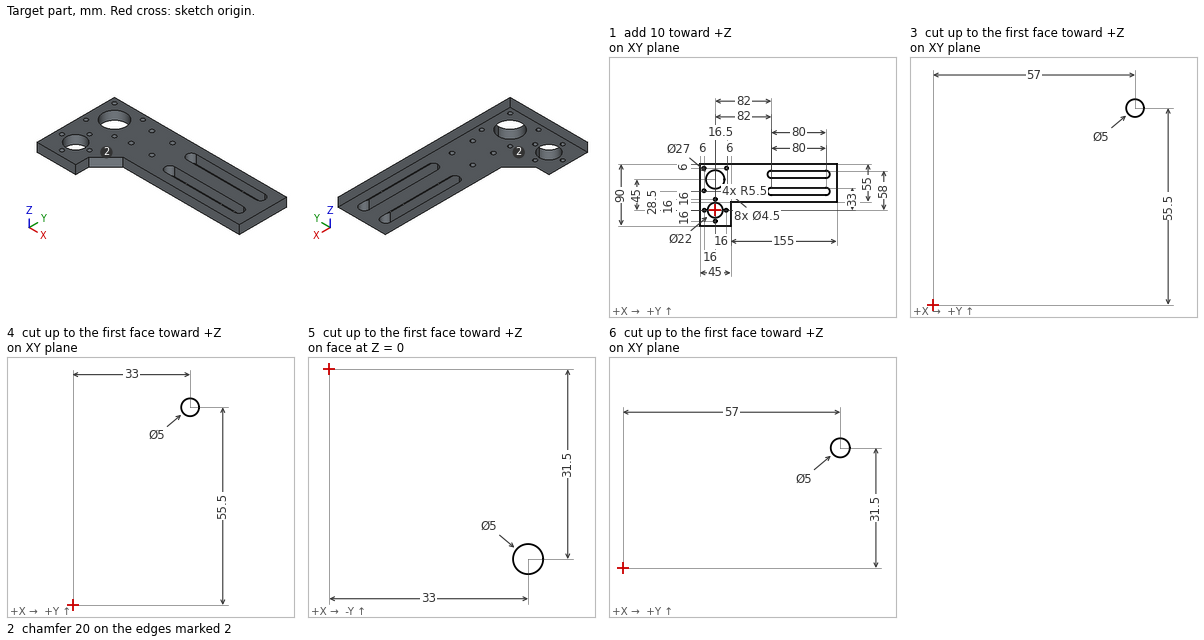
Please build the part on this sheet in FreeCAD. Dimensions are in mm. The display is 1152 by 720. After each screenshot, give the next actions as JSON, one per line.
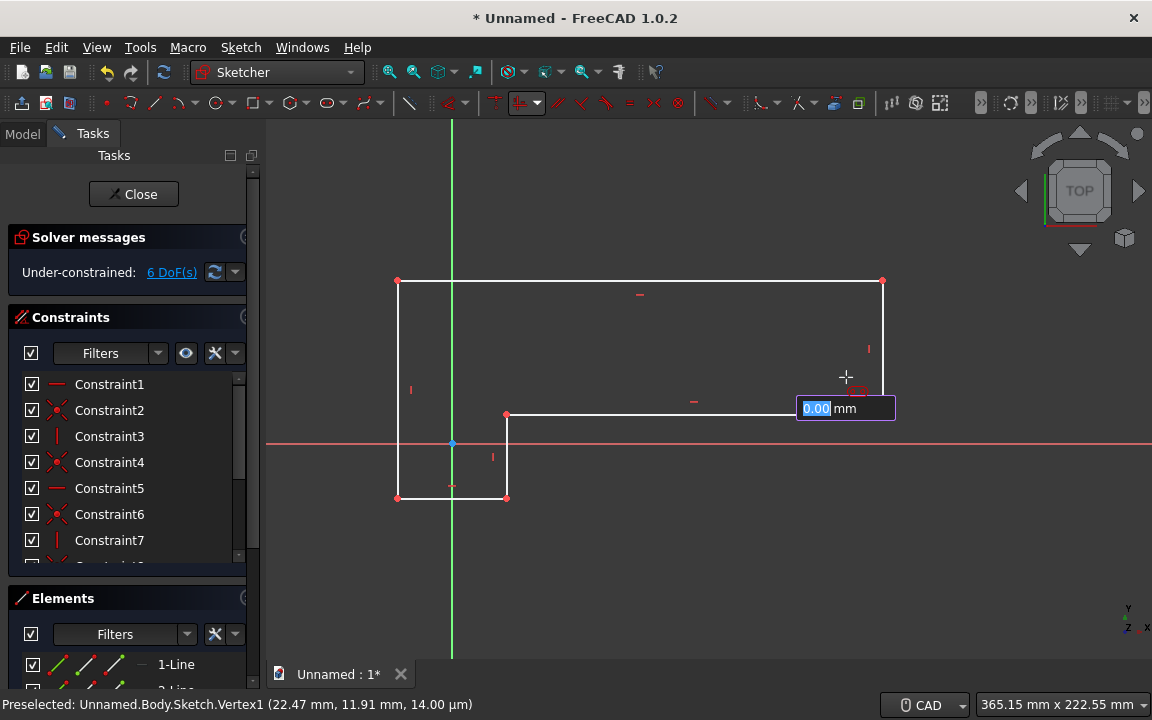
{"action": "left_click", "coordinate": [749, 391]}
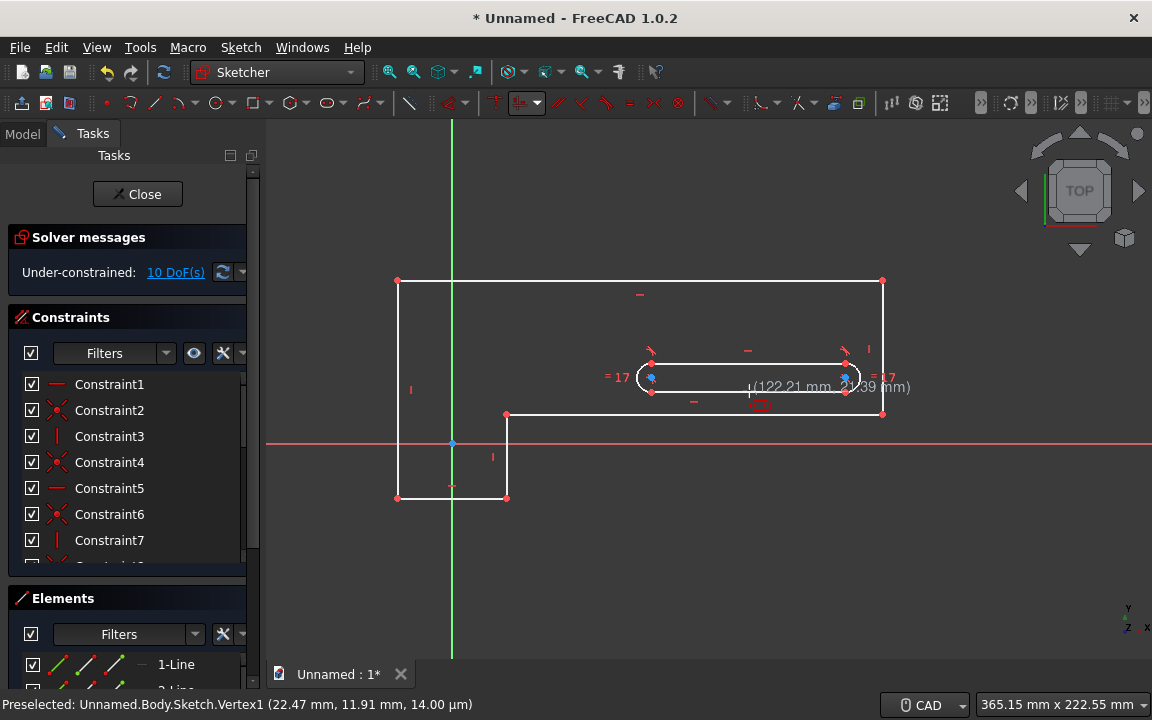
{"action": "scroll", "coordinate": [651, 317], "scroll_direction": "up", "scroll_amount": 3}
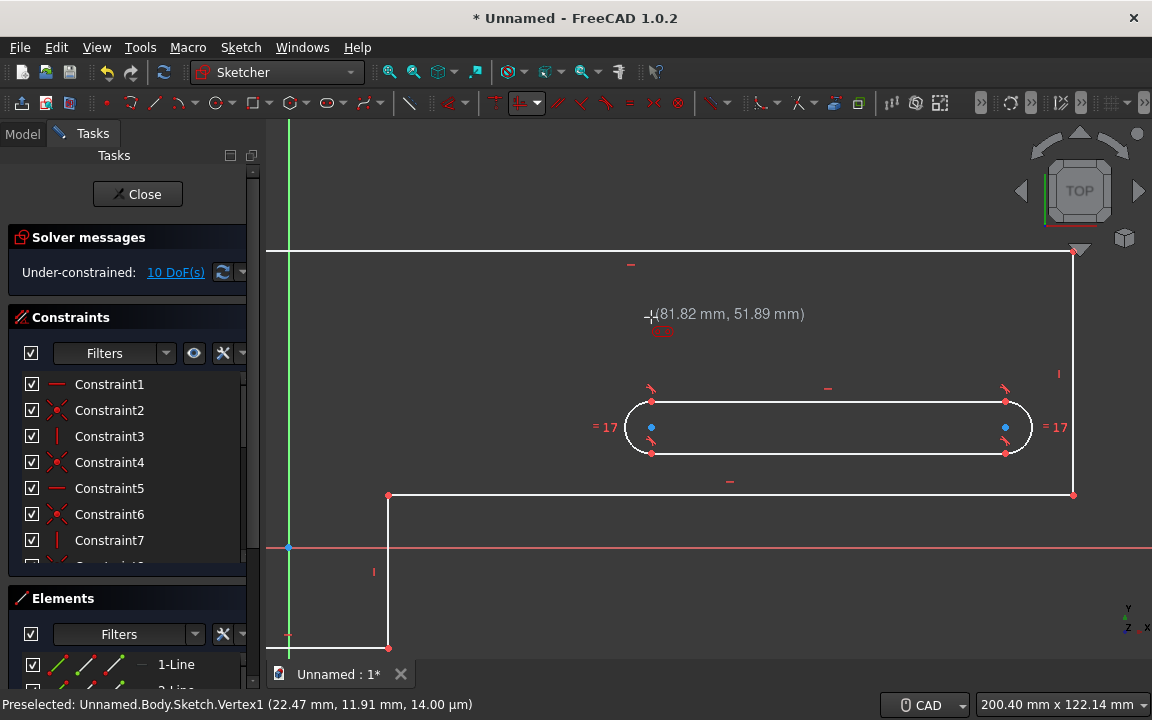
{"action": "left_click", "coordinate": [651, 316]}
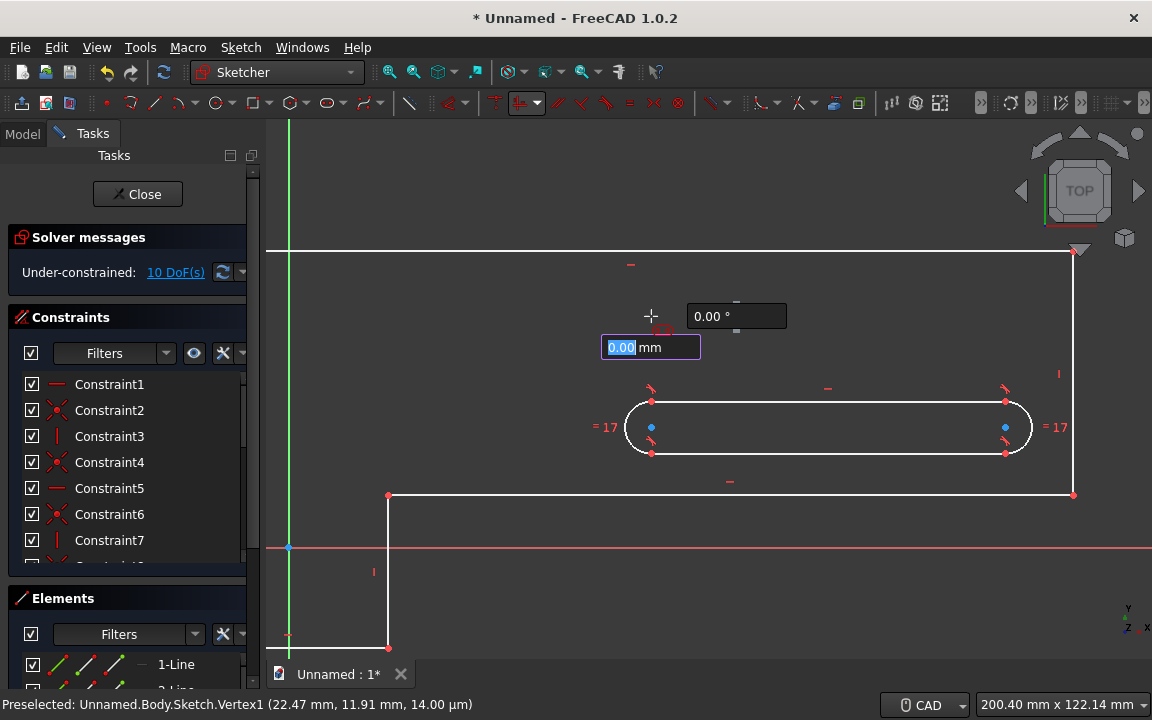
{"action": "scroll", "coordinate": [651, 317], "scroll_direction": "down", "scroll_amount": 3}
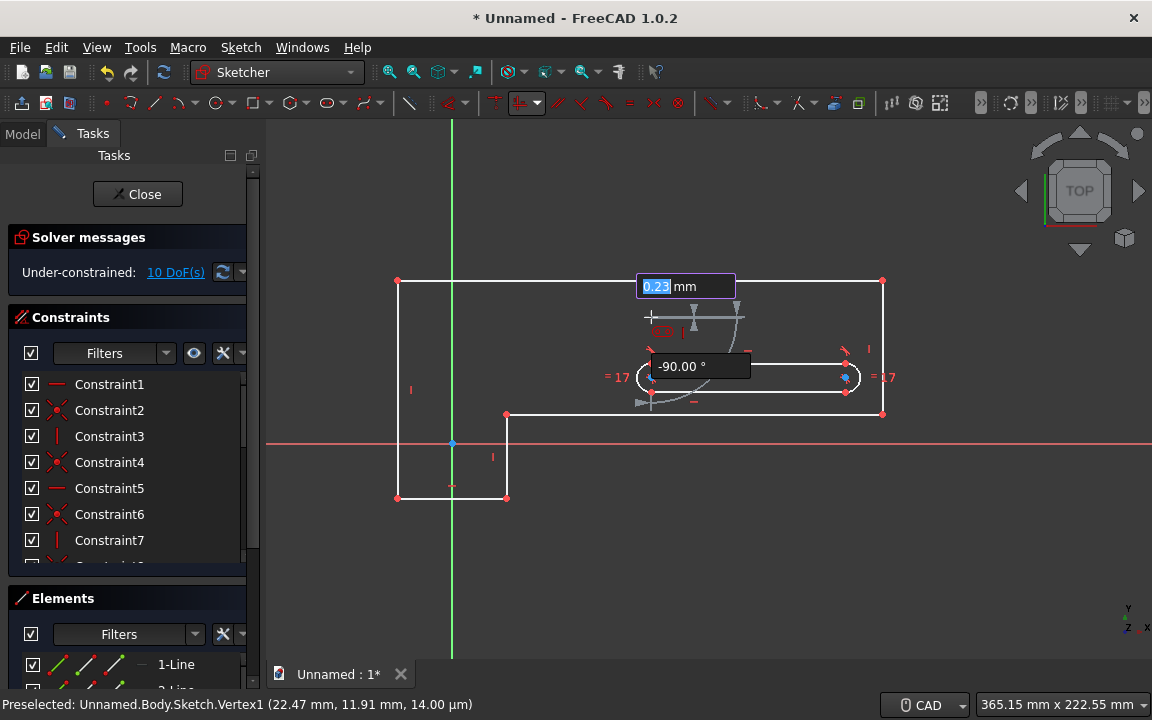
{"action": "left_click", "coordinate": [846, 317]}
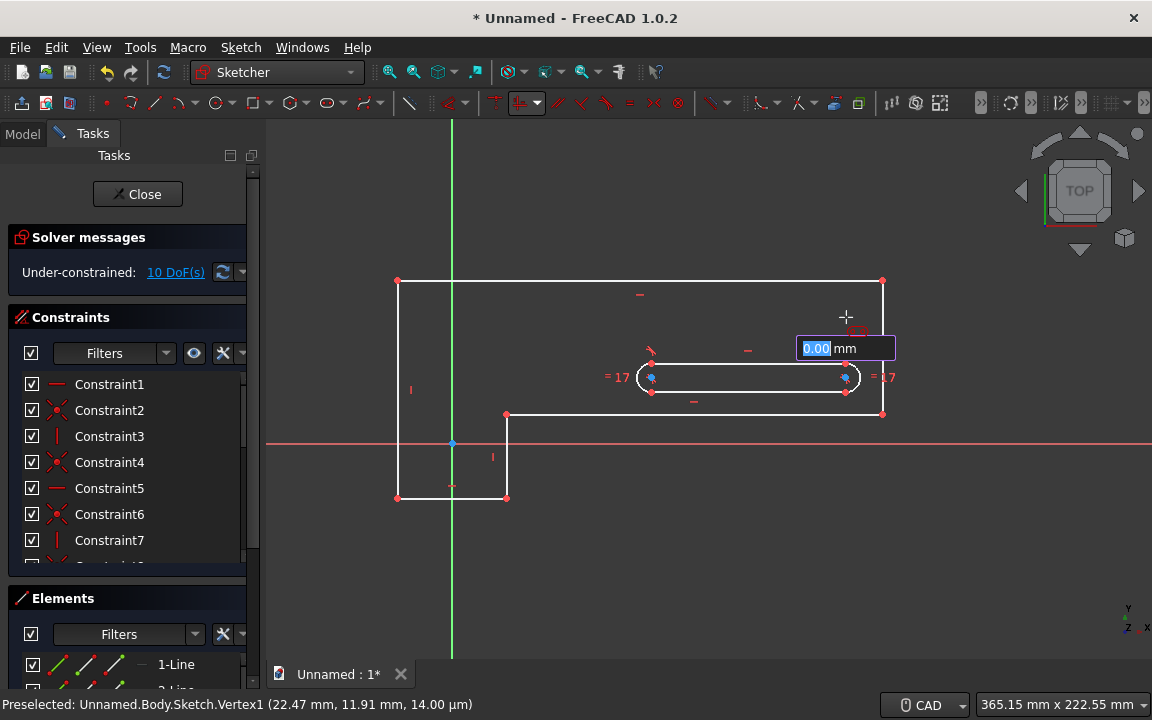
{"action": "left_click", "coordinate": [749, 330]}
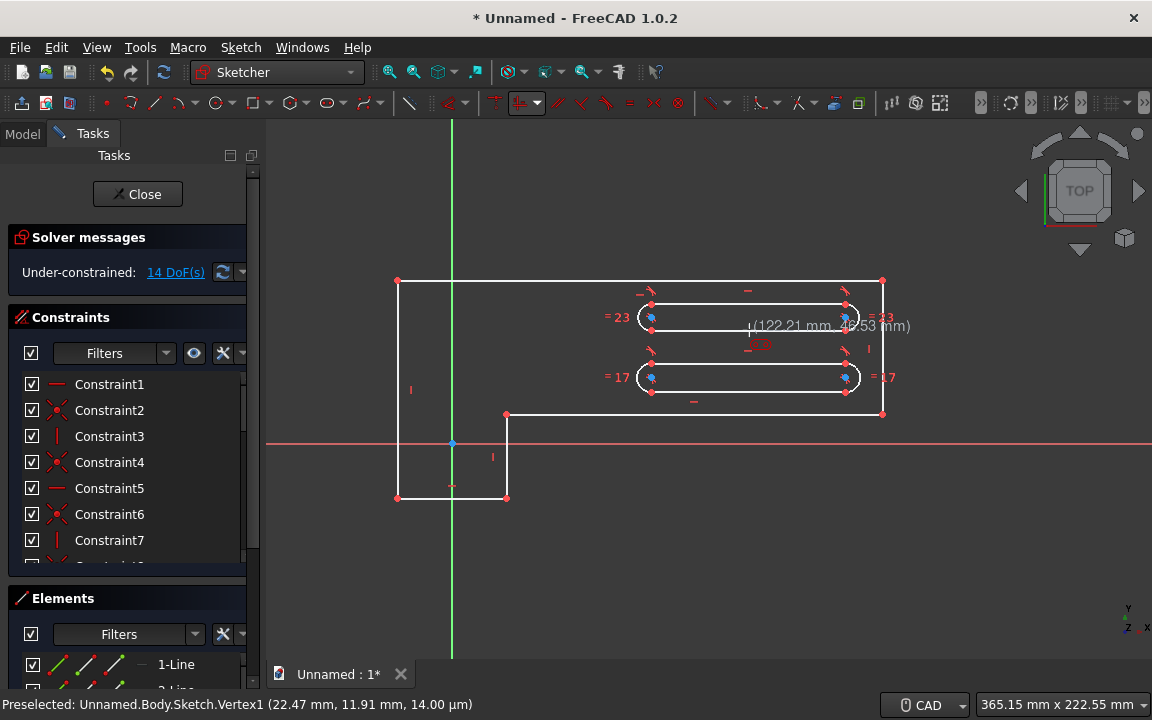
{"action": "key", "text": "g c"}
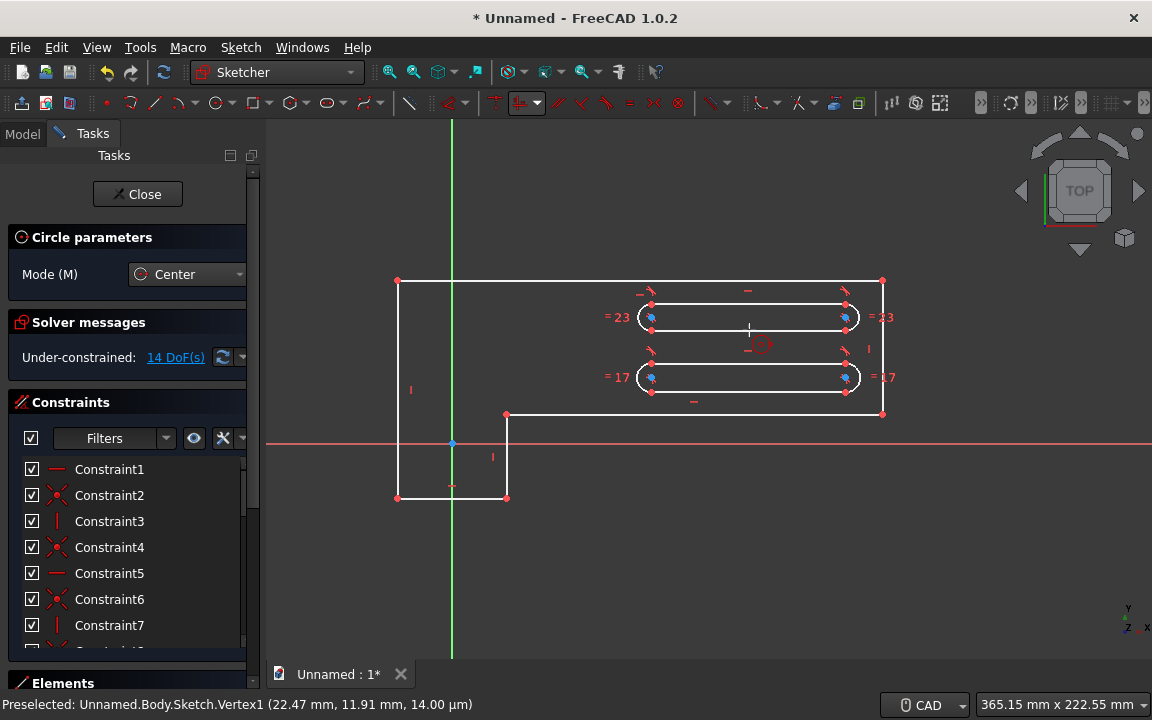
{"action": "scroll", "coordinate": [452, 483], "scroll_direction": "up", "scroll_amount": 8}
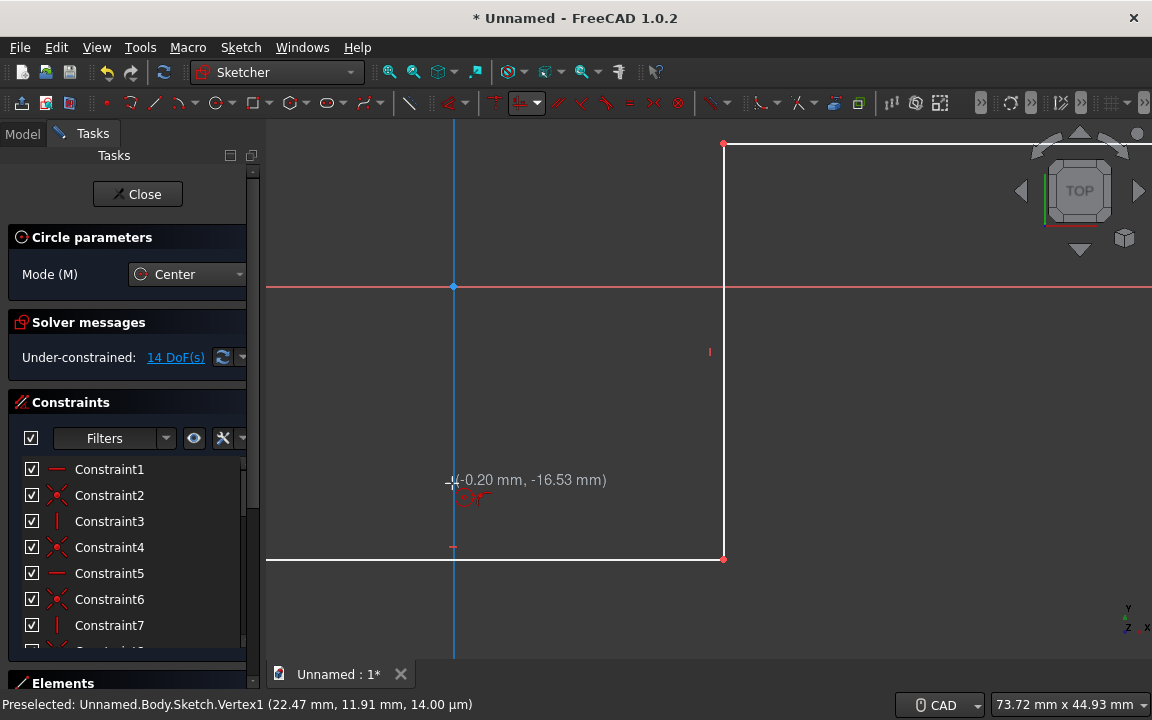
{"action": "scroll", "coordinate": [452, 483], "scroll_direction": "down", "scroll_amount": 8}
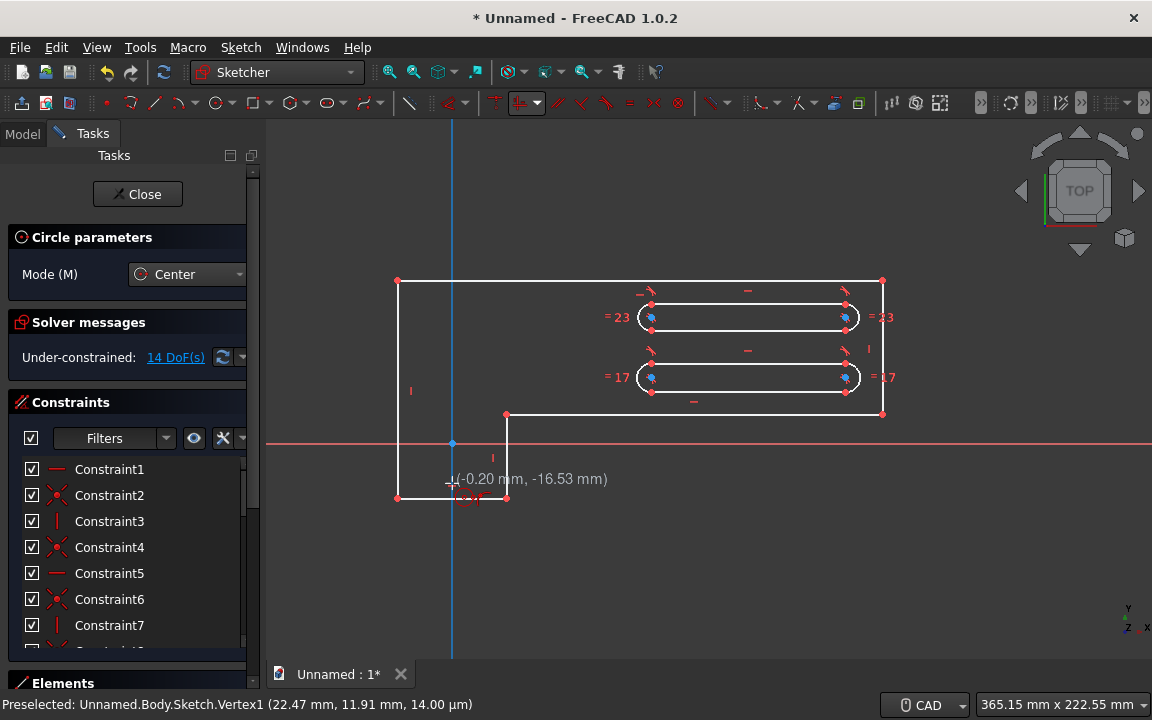
{"action": "left_click", "coordinate": [452, 483]}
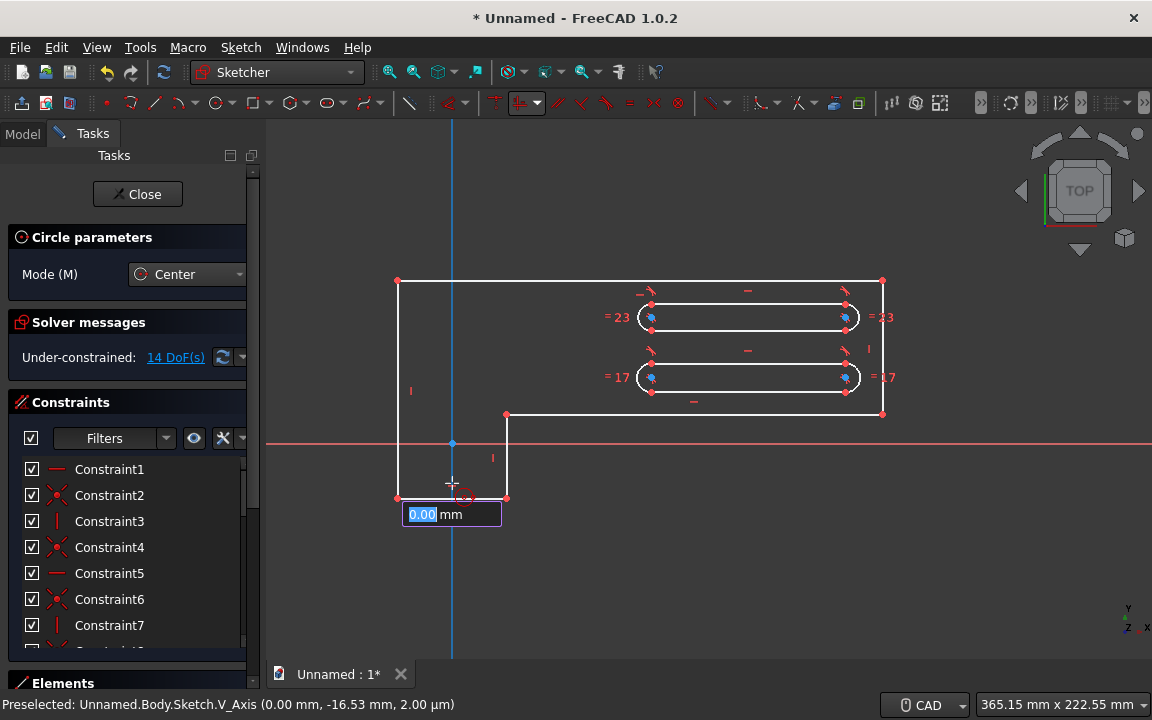
{"action": "scroll", "coordinate": [458, 481], "scroll_direction": "up", "scroll_amount": 6}
{"action": "mouse_move", "coordinate": [456, 479]}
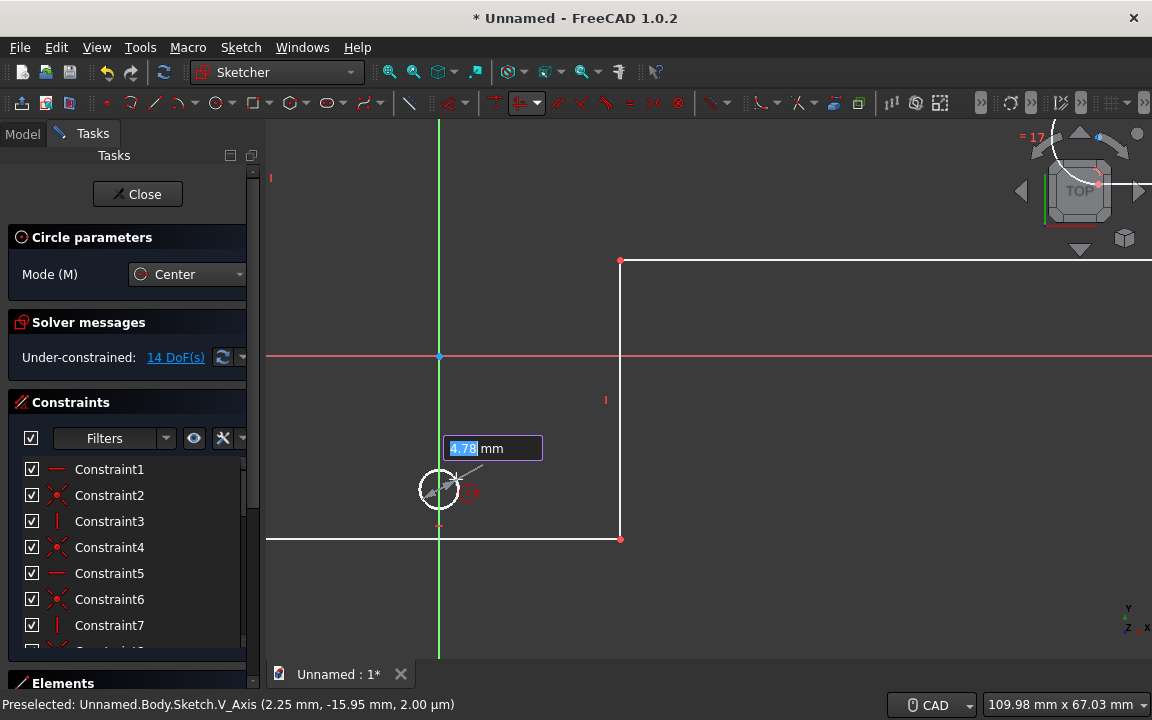
{"action": "type", "text": "4.5"}
{"action": "key", "text": "Return"}